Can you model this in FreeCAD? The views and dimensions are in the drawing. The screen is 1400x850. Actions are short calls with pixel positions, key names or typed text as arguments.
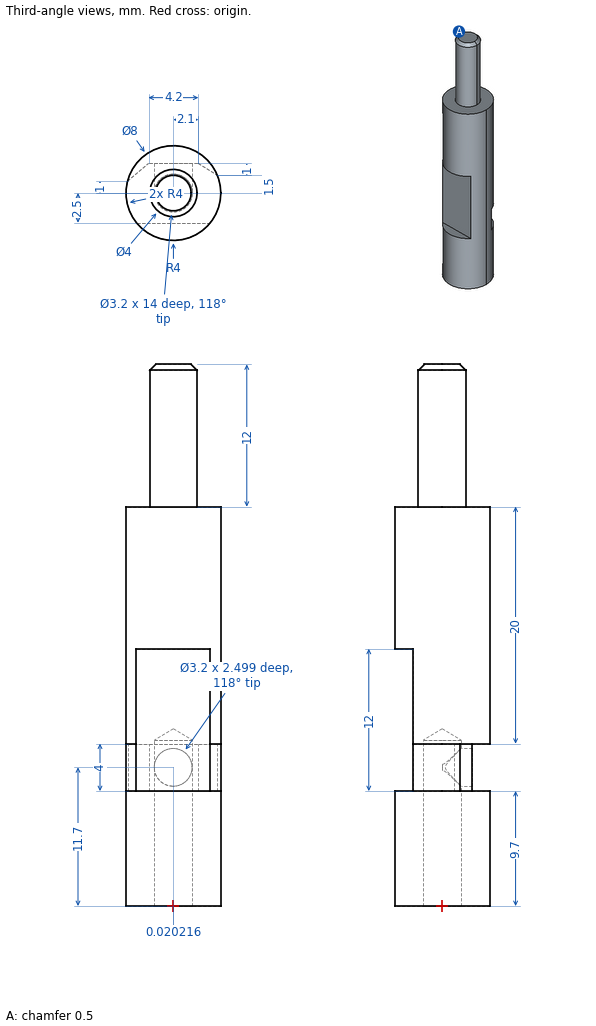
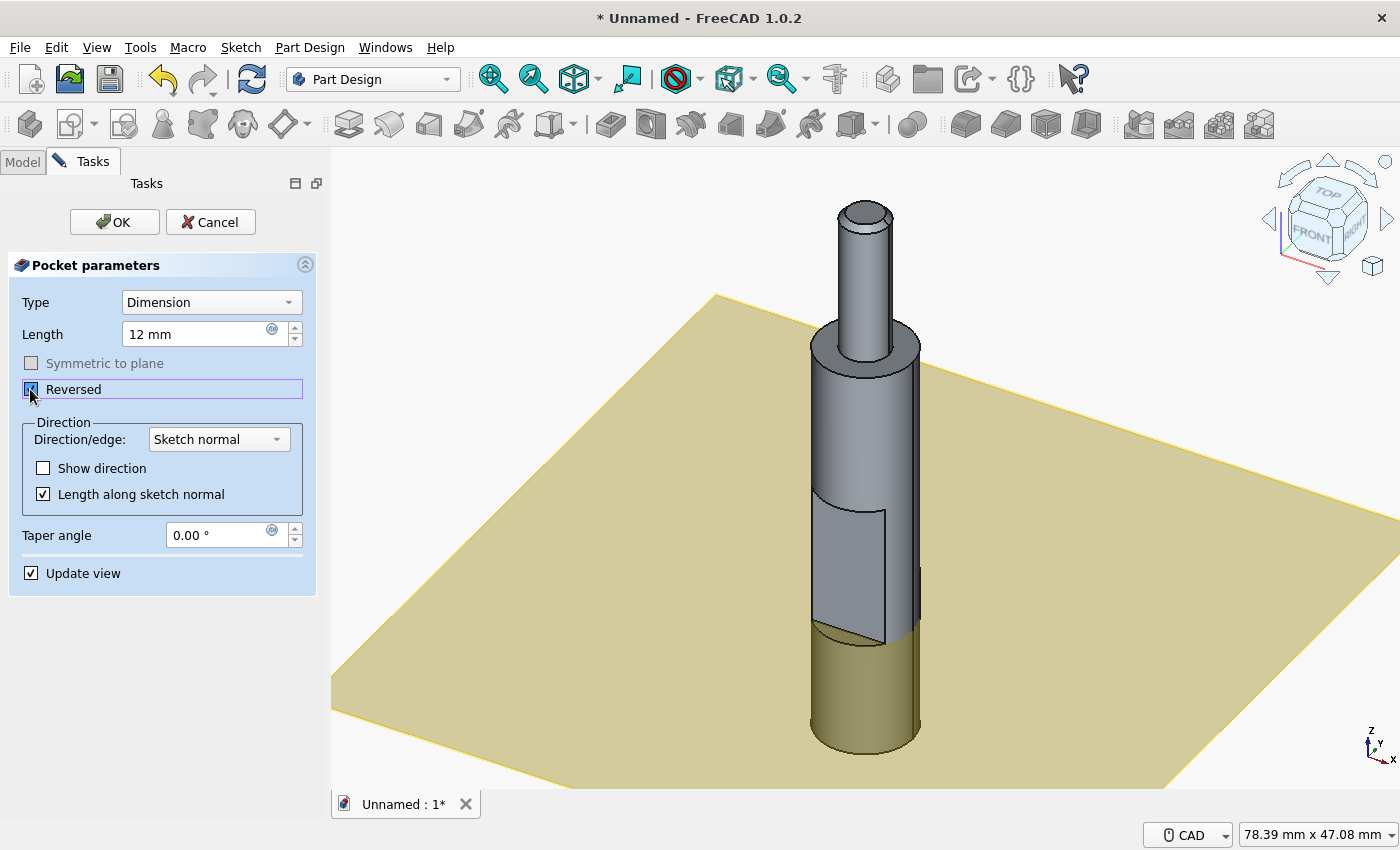
click(115, 222)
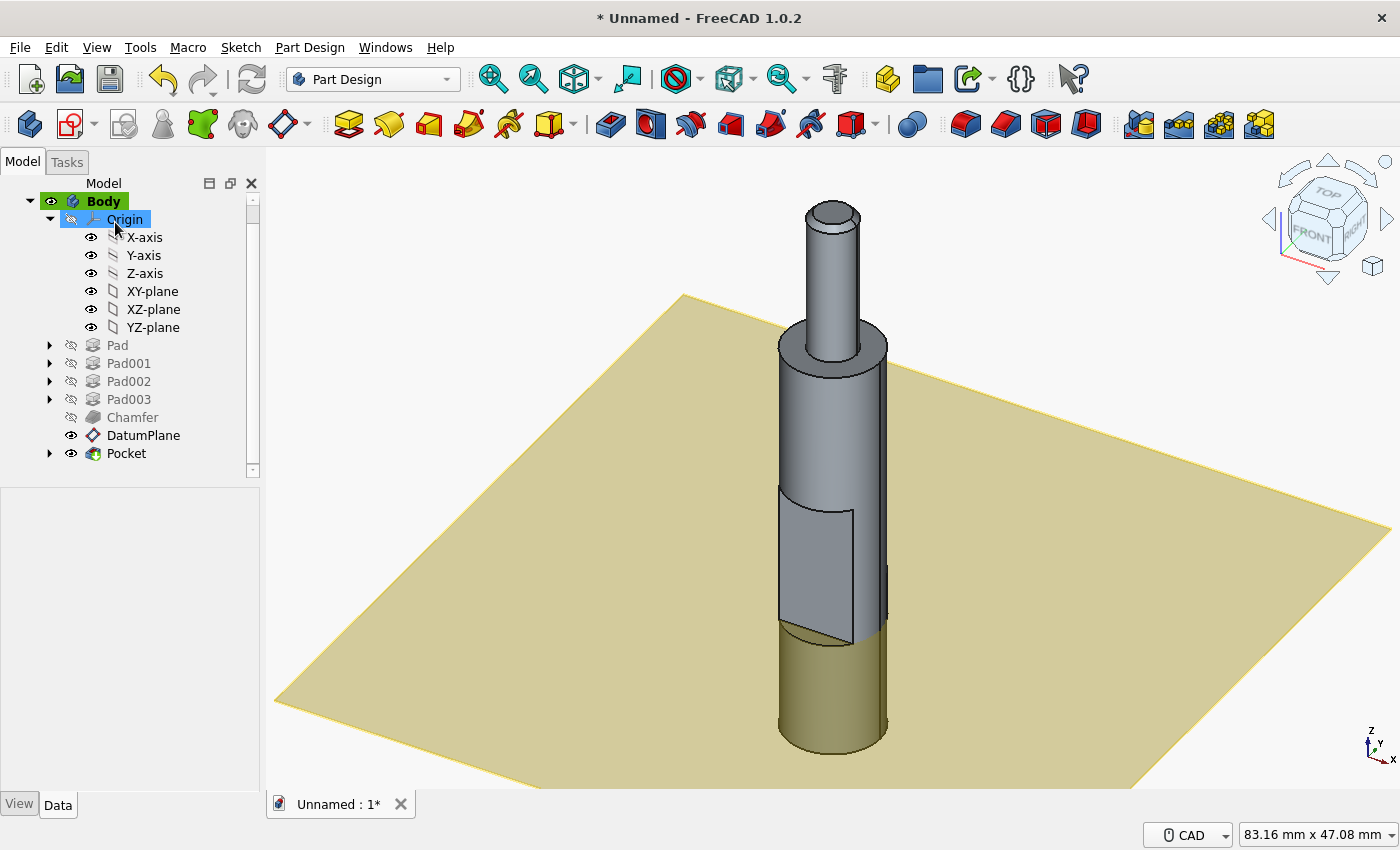
click(116, 435)
key(space)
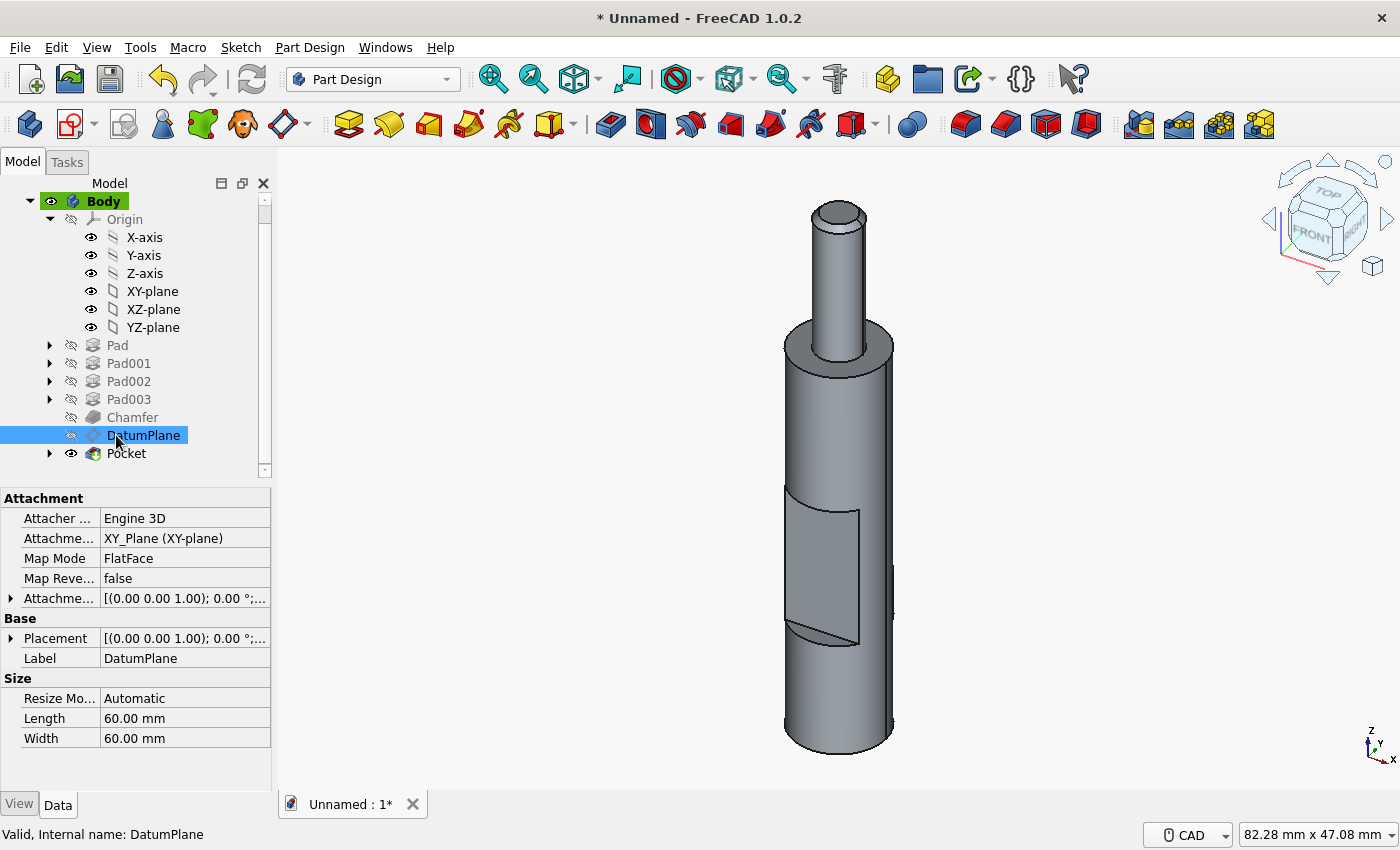
key(5)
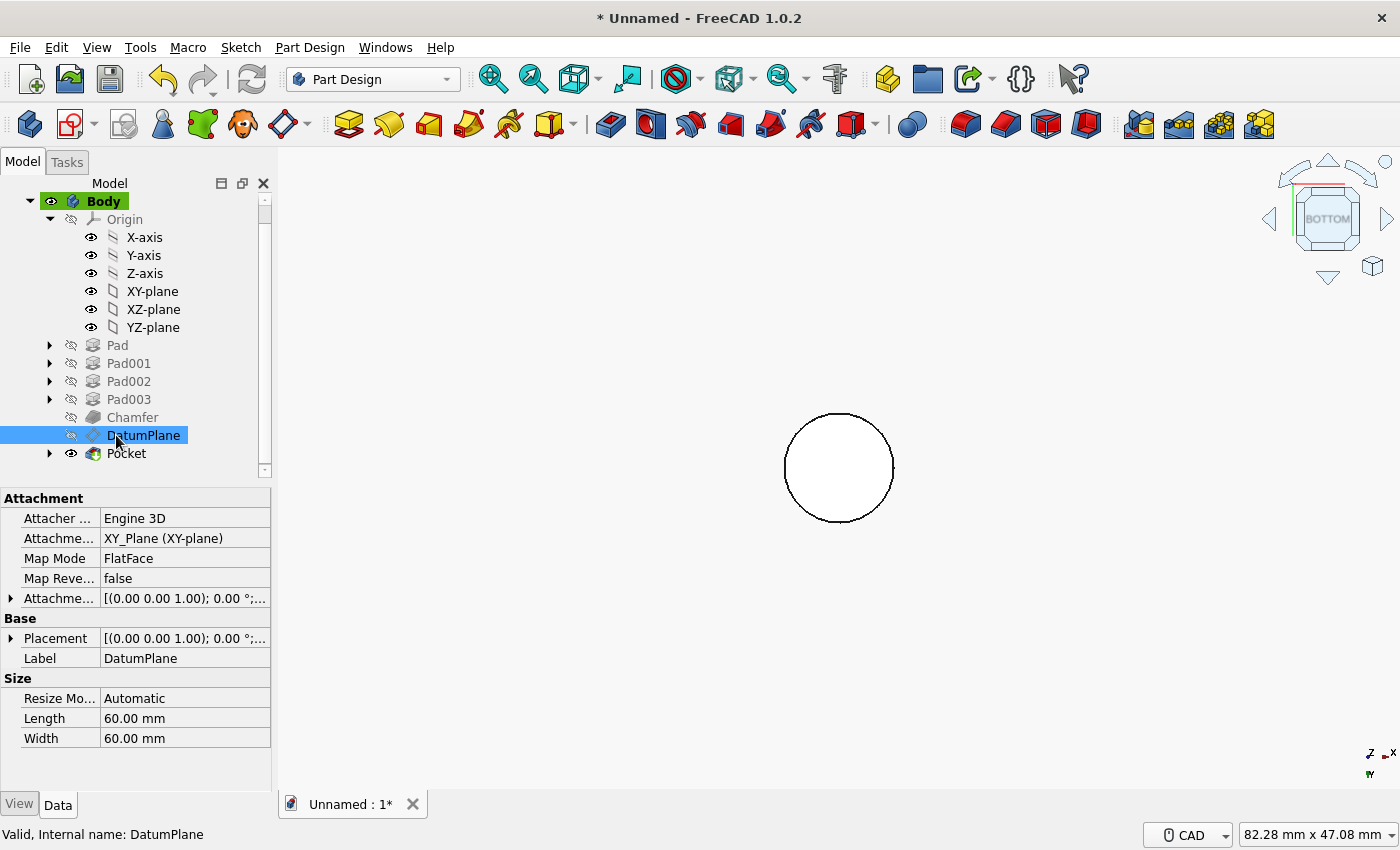
key(v)
key(f)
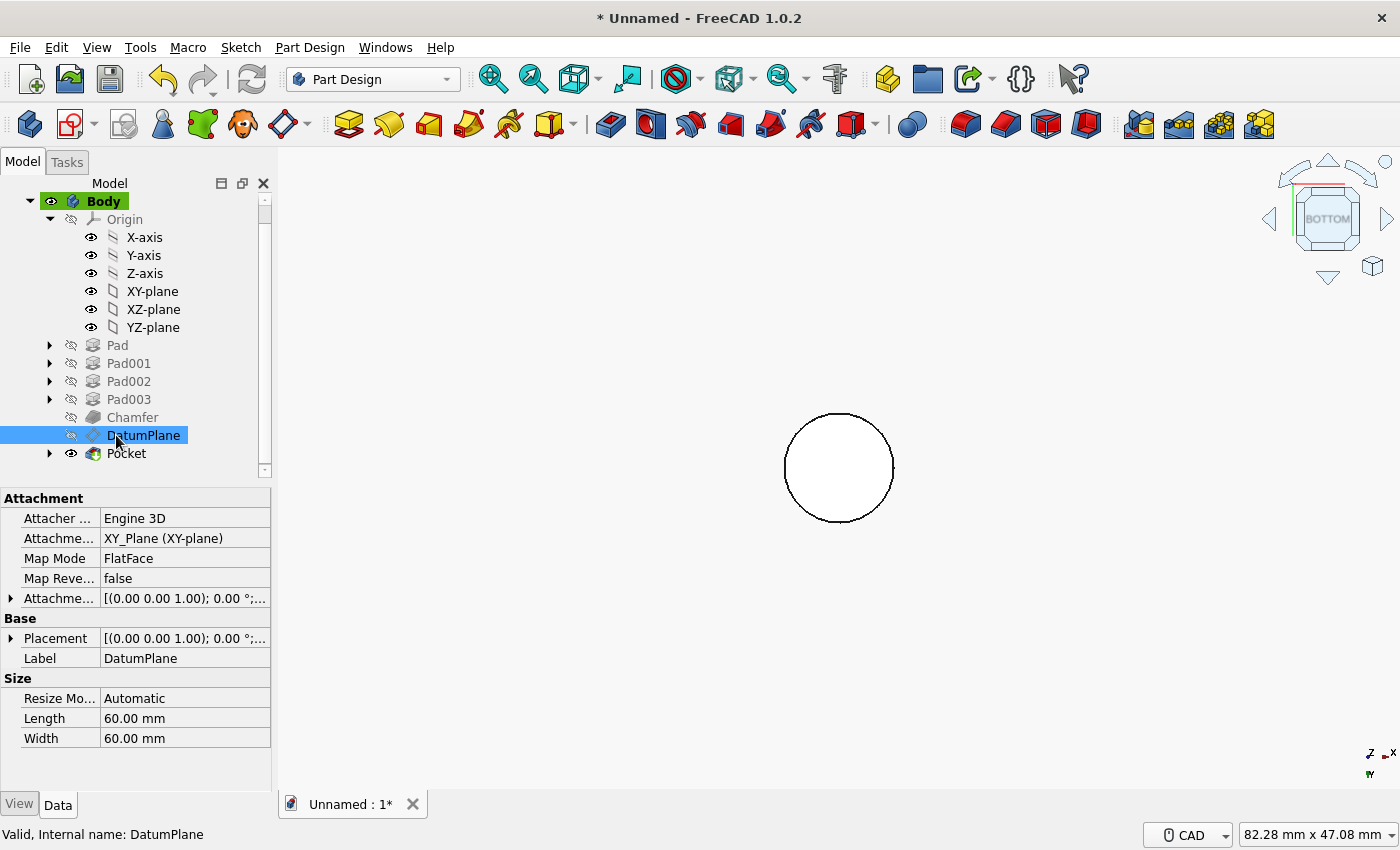
click(839, 467)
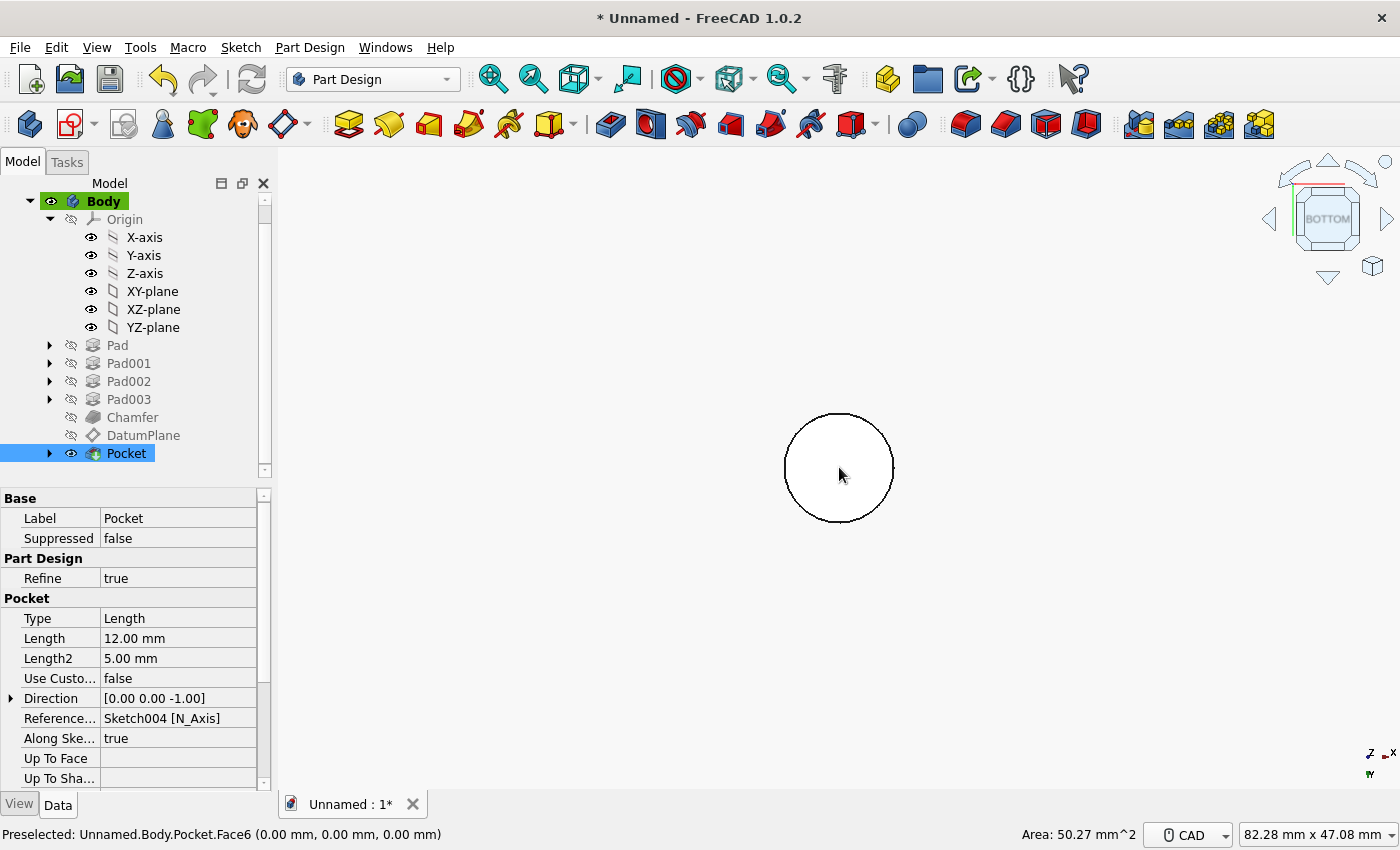
click(70, 124)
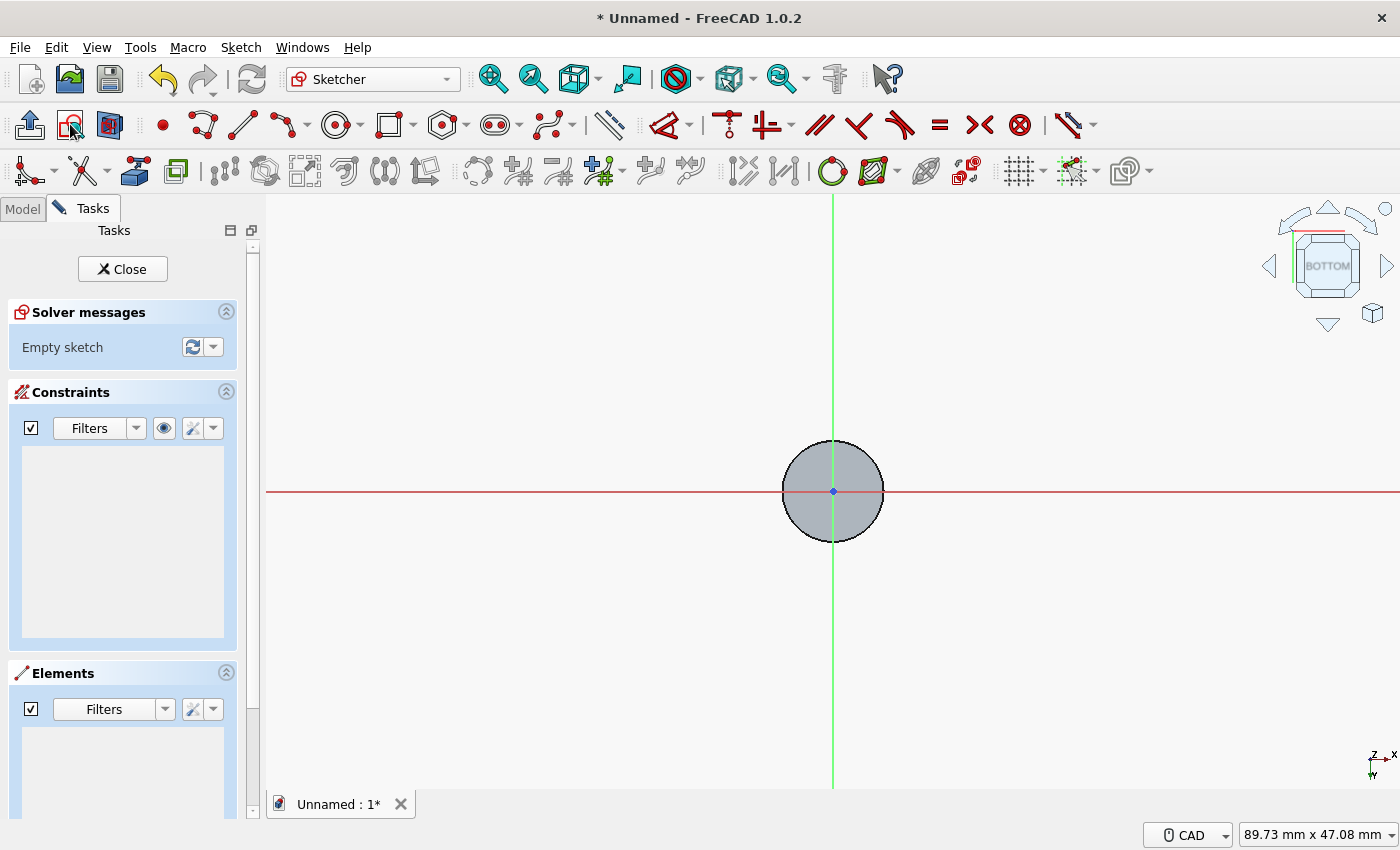
scroll(842, 492, up, 11)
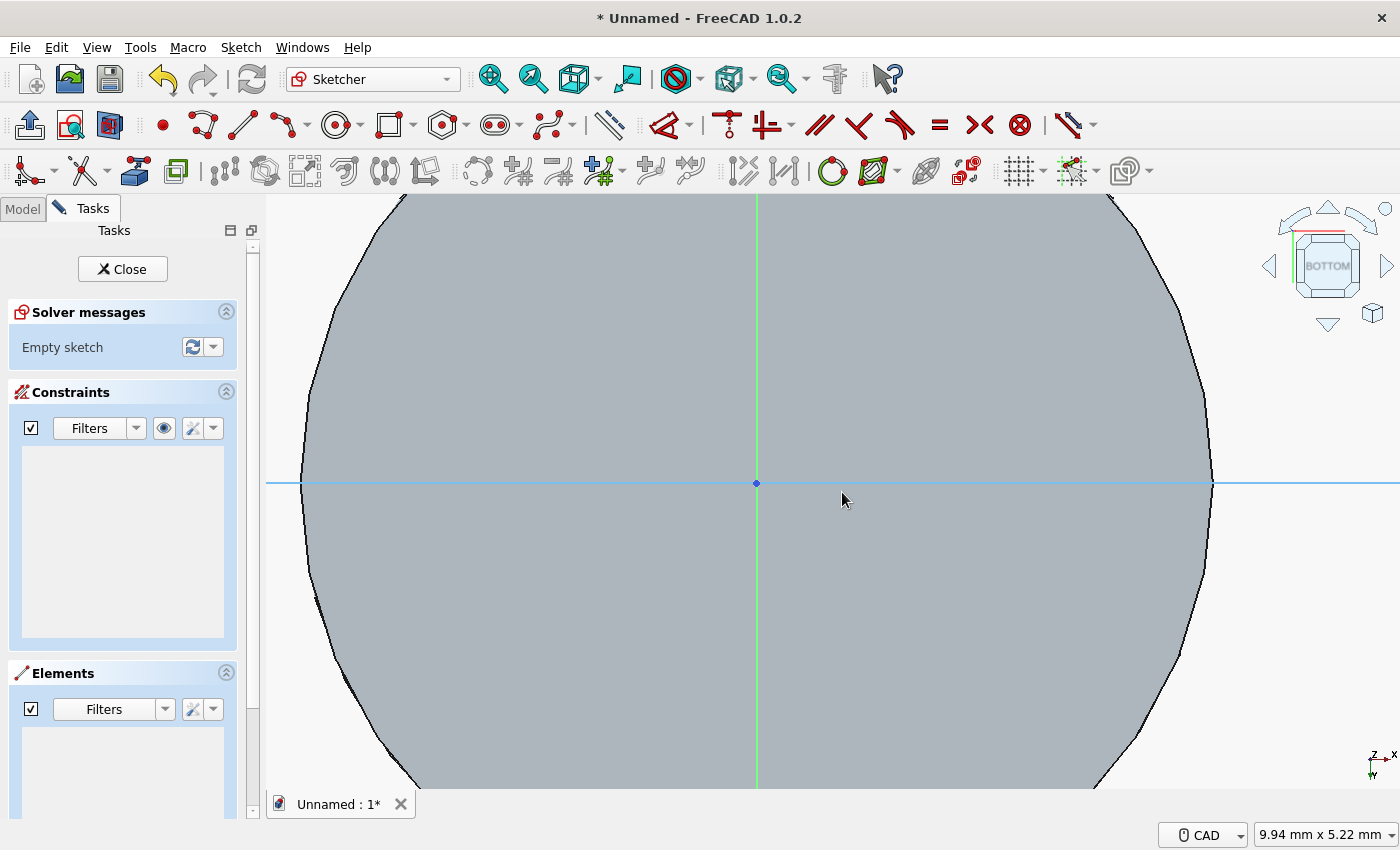
key(g)
key(c)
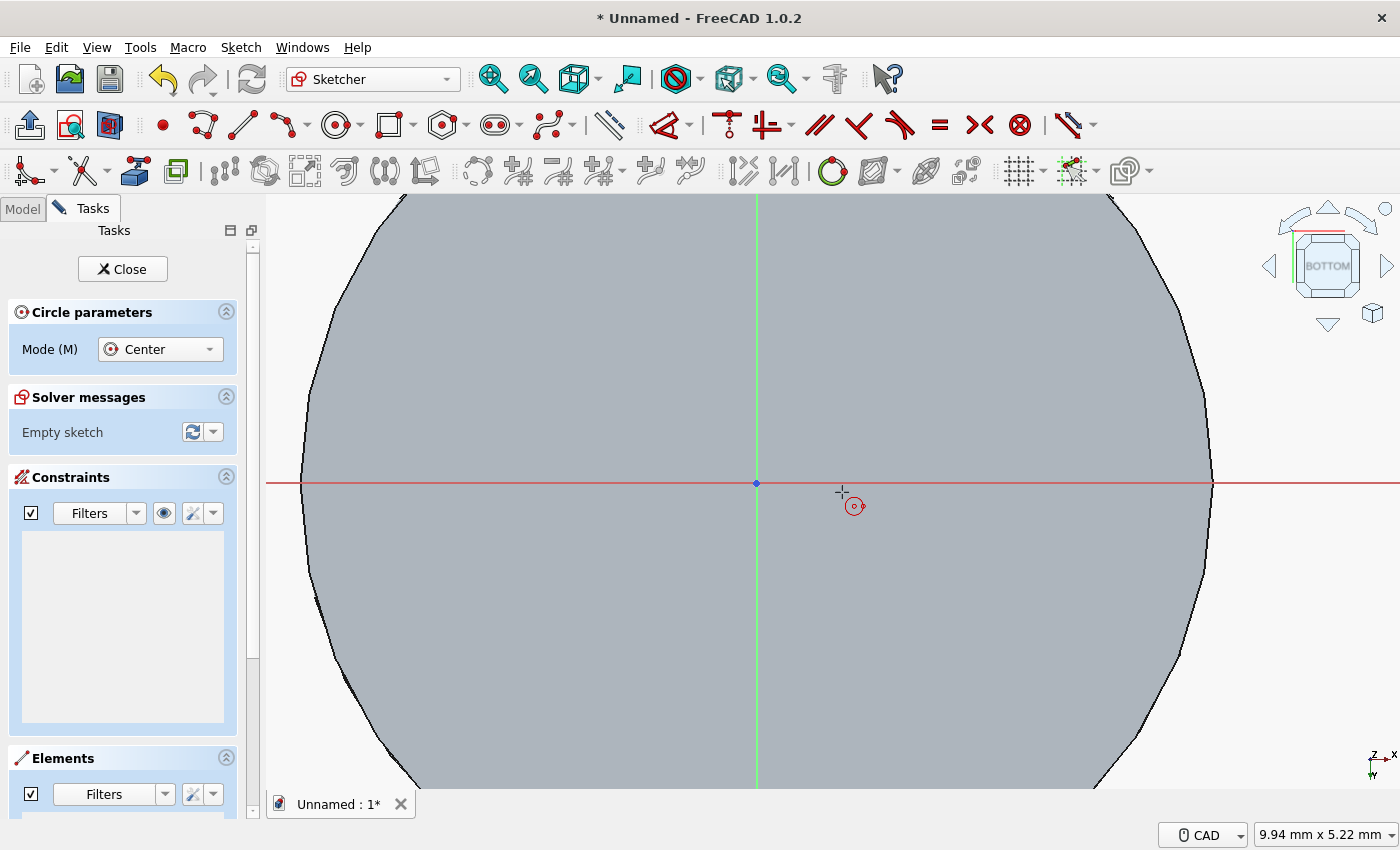
click(757, 483)
click(886, 354)
key(Escape)